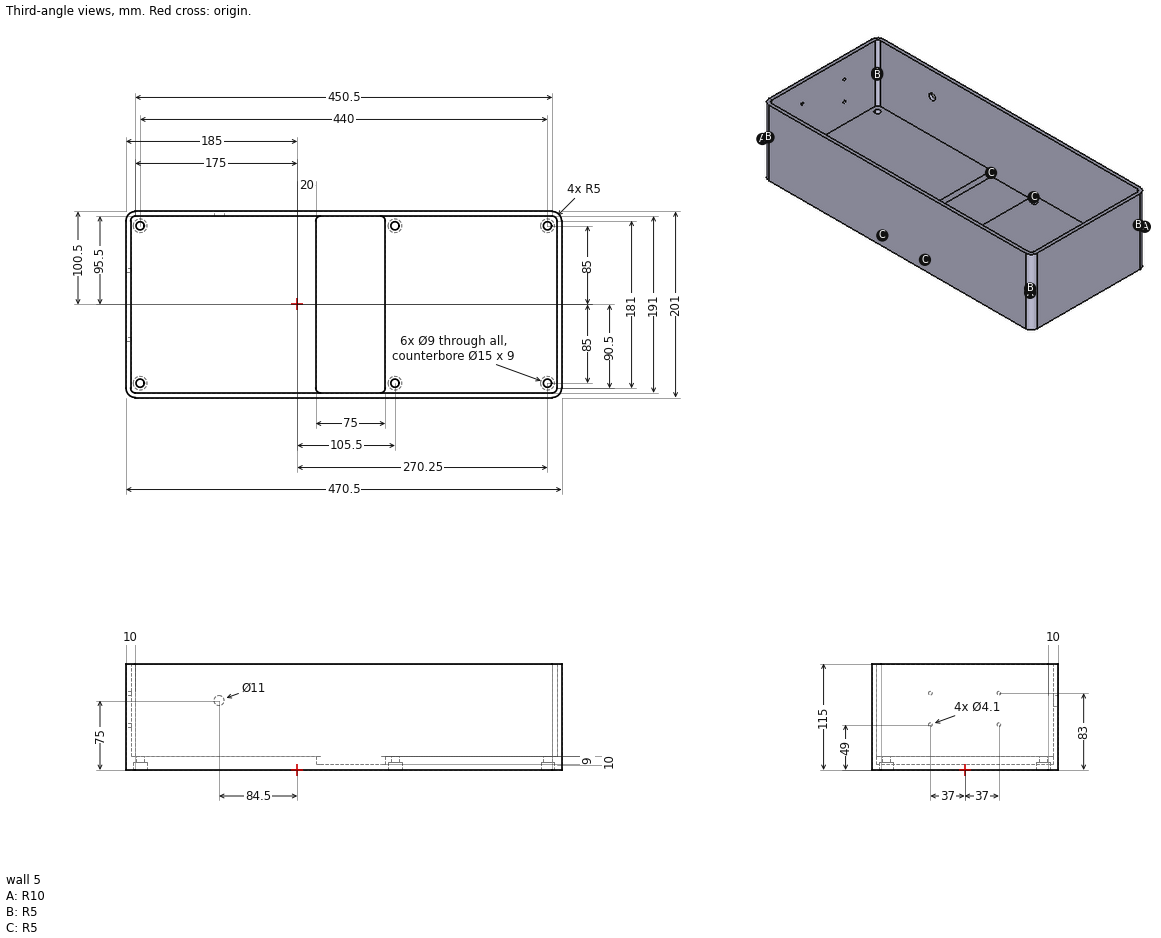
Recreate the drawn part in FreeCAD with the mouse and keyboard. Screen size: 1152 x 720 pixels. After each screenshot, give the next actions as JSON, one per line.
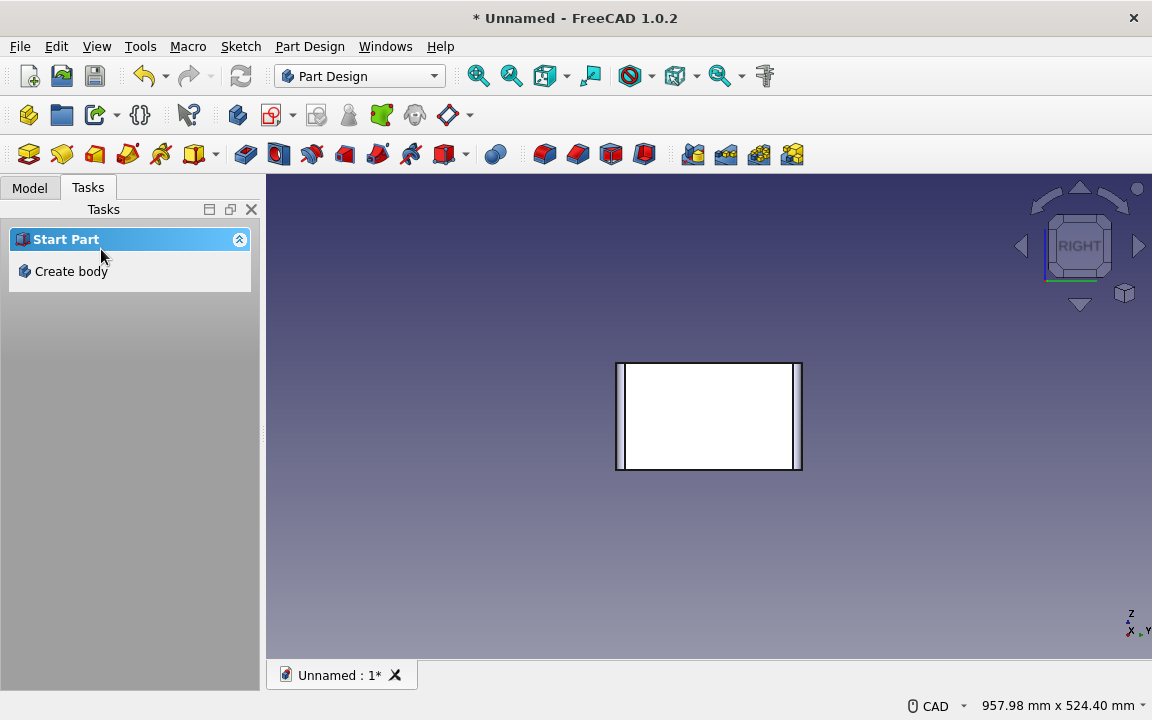
{"action": "key", "text": "5"}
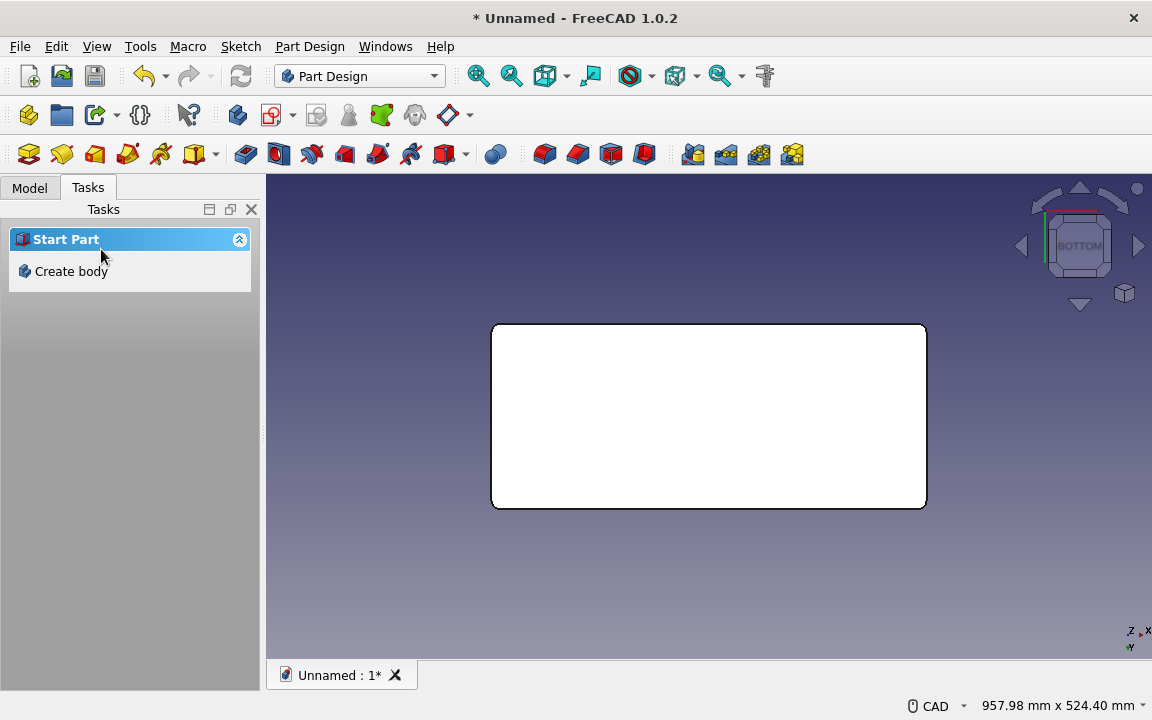
{"action": "key", "text": "4"}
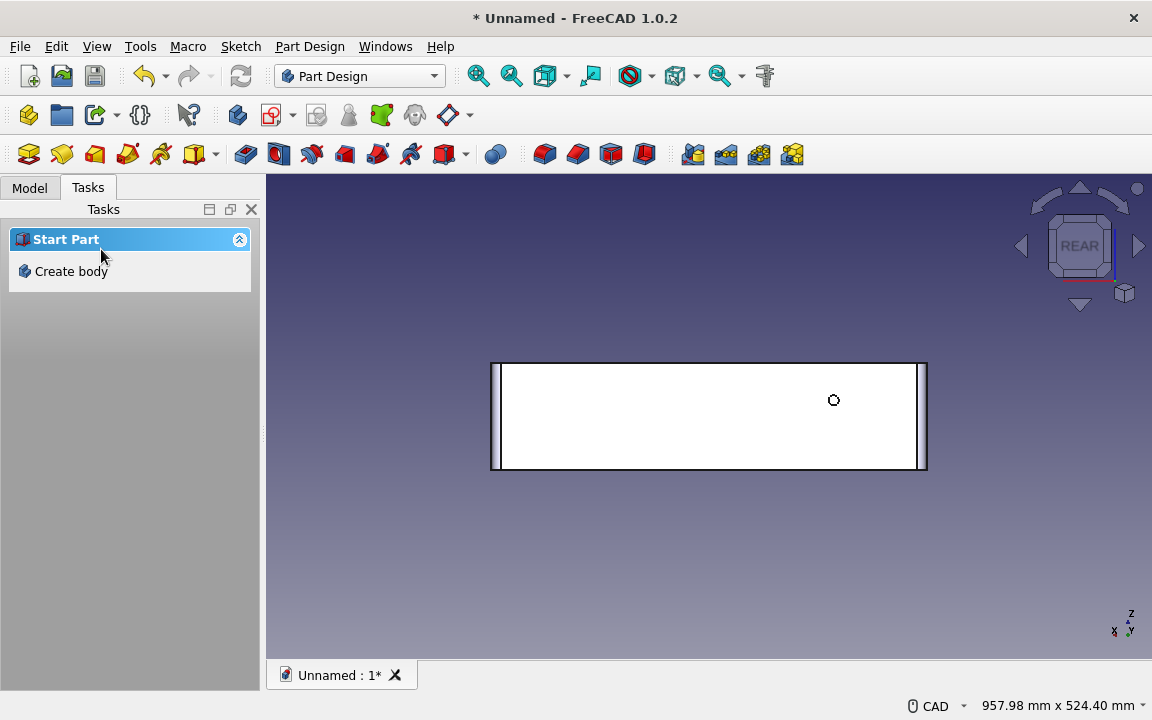
{"action": "key", "text": "6"}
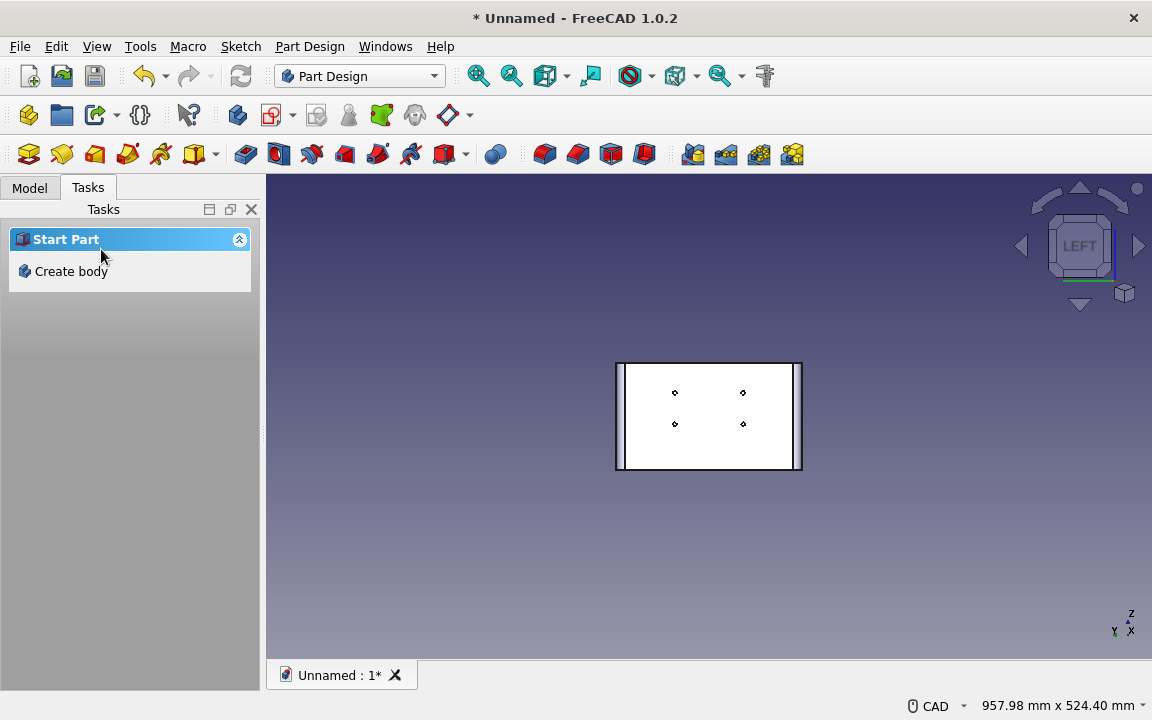
{"action": "key", "text": "v f"}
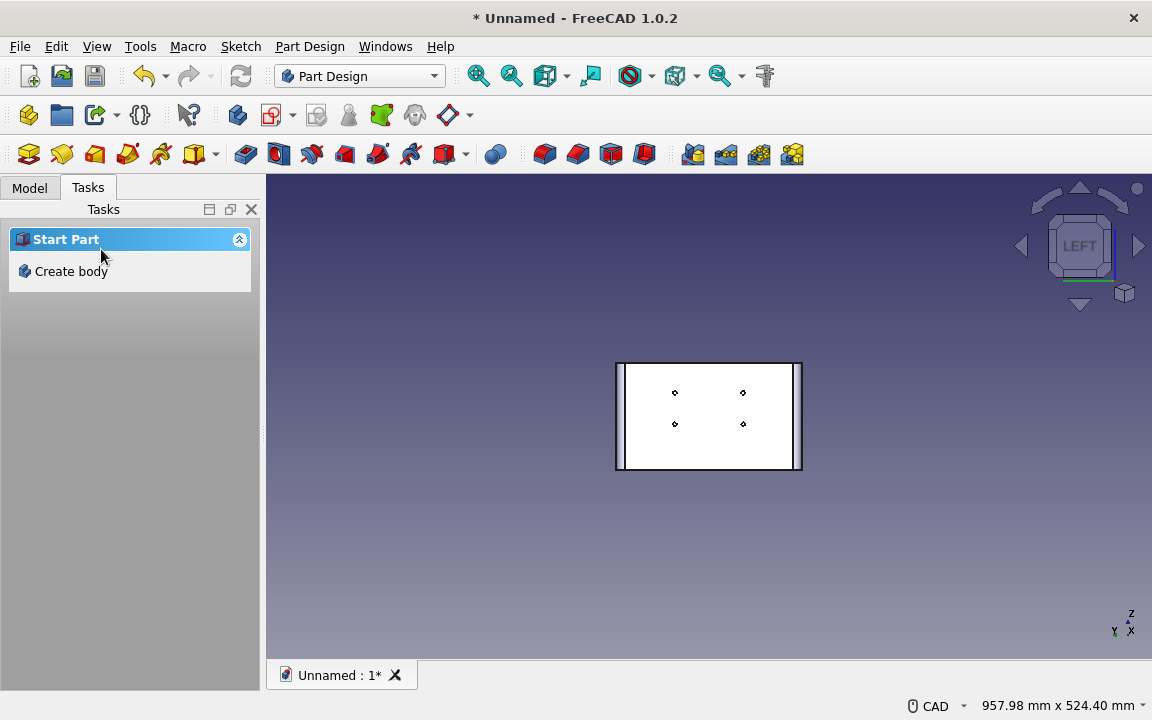
{"action": "key", "text": "v 3"}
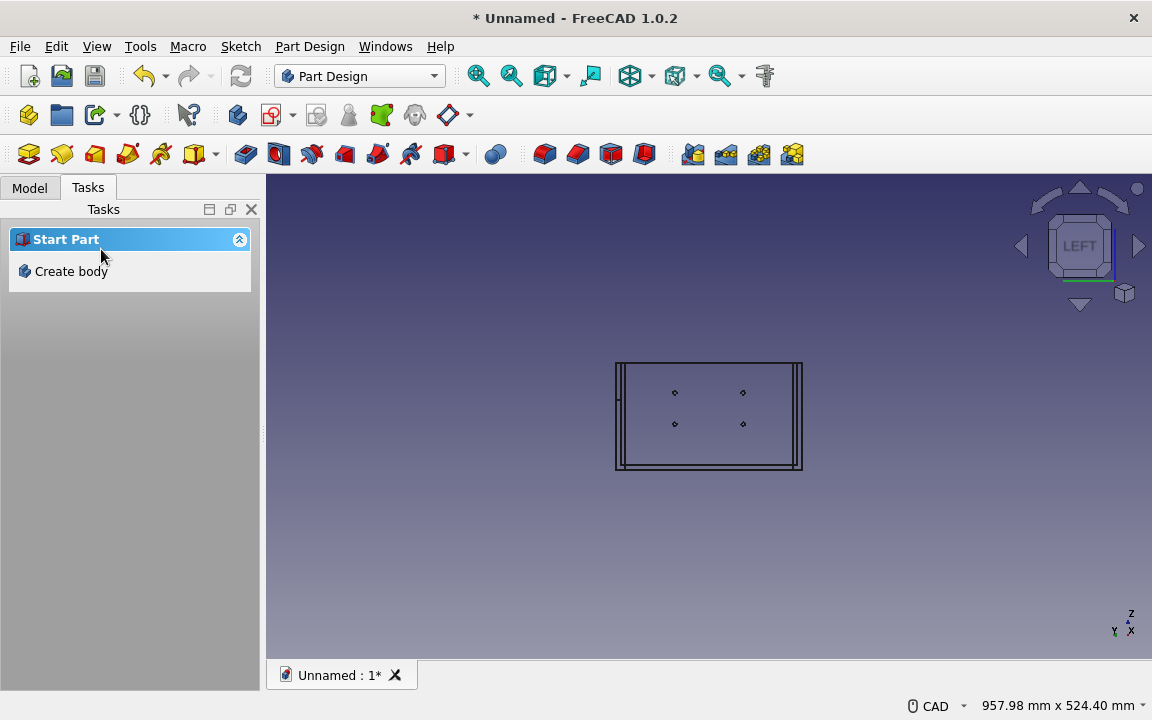
{"action": "key", "text": "0"}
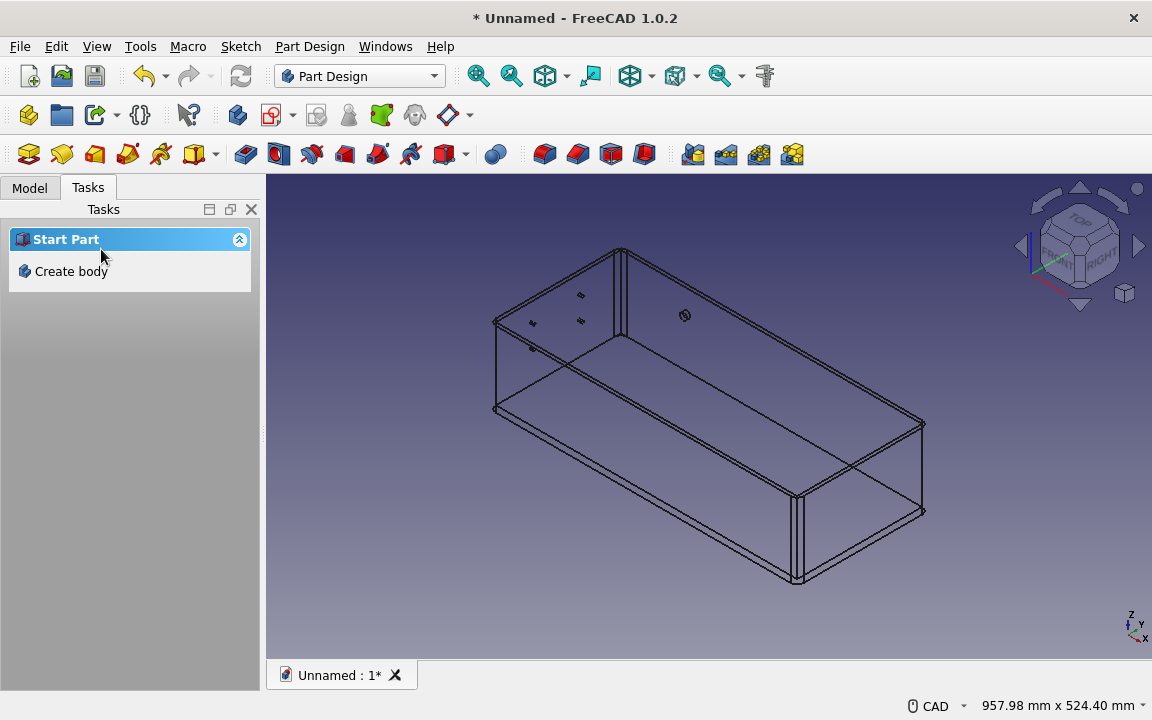
{"action": "left_click", "coordinate": [797, 537]}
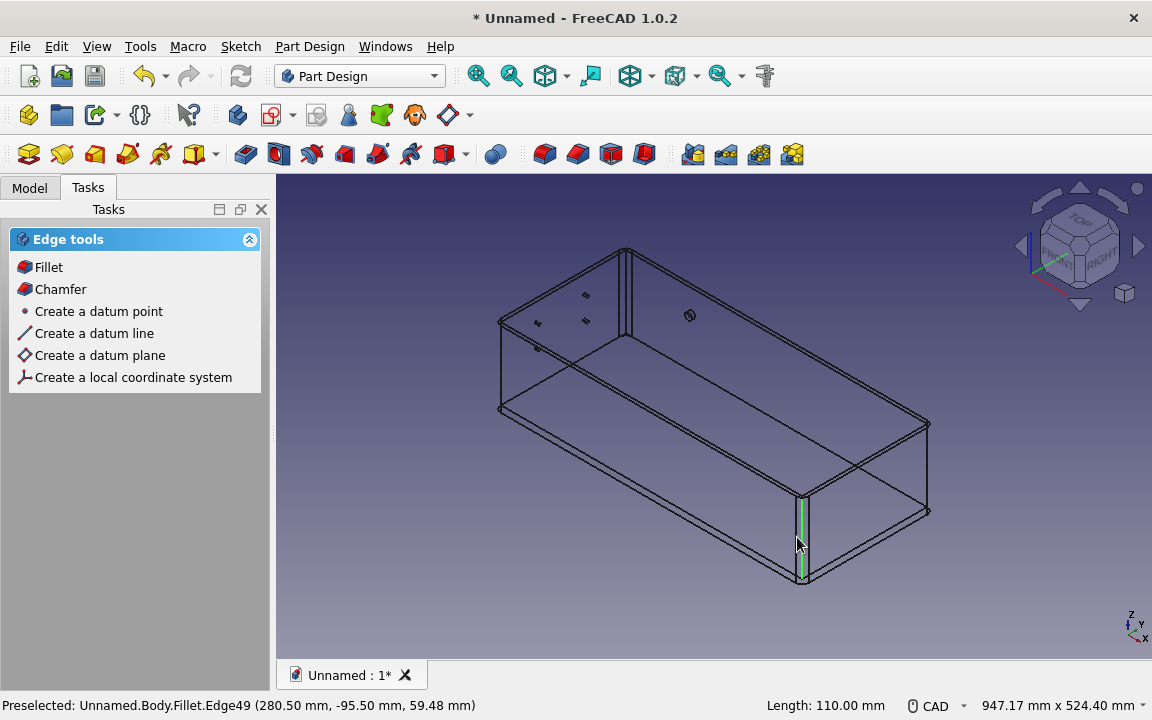
{"action": "left_click", "coordinate": [626, 291], "text": "ctrl"}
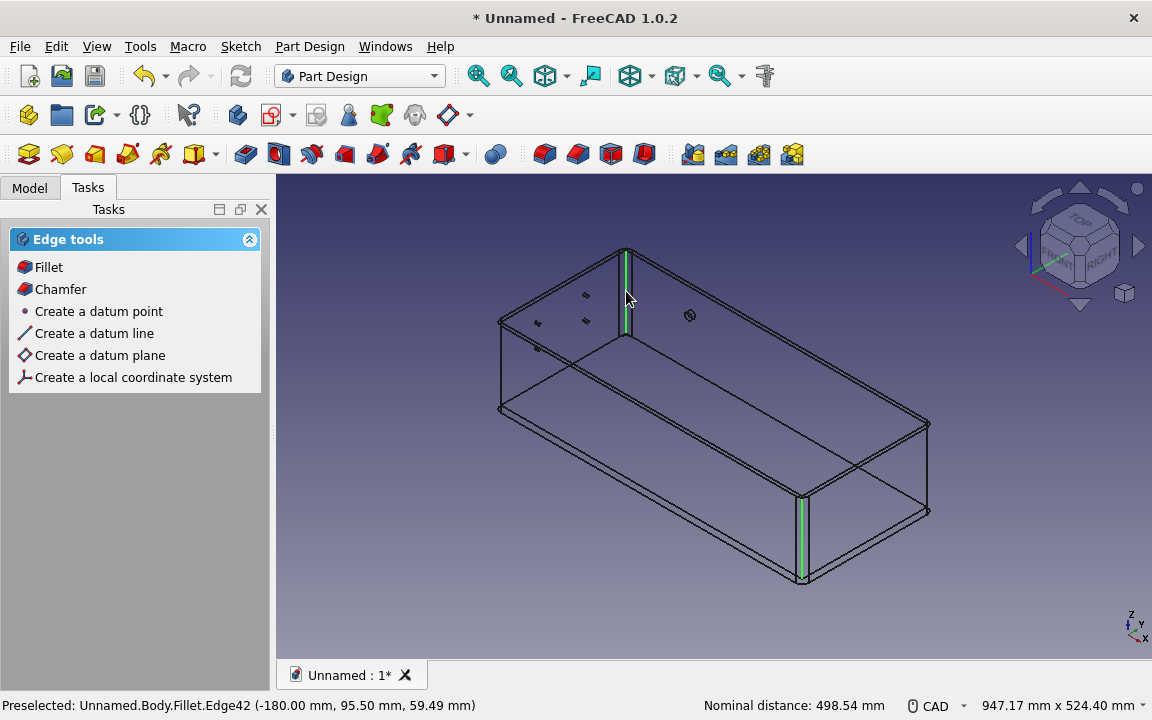
{"action": "scroll", "coordinate": [927, 464], "scroll_direction": "up", "scroll_amount": 6}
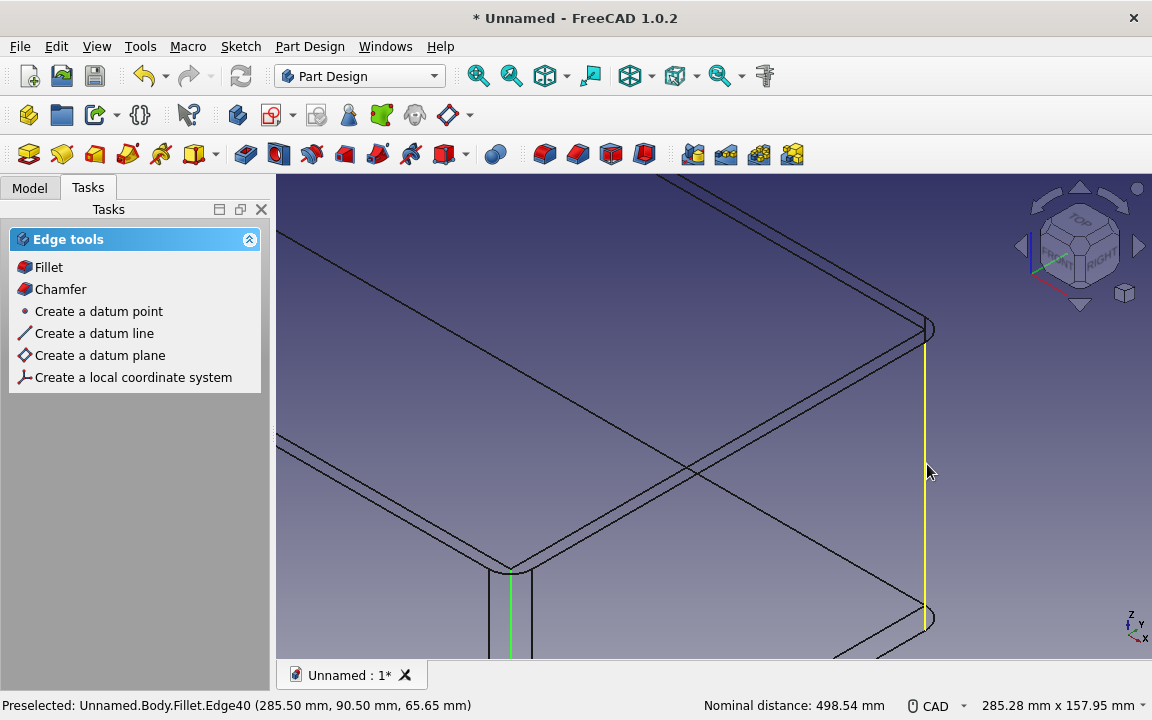
{"action": "left_click", "coordinate": [479, 76]}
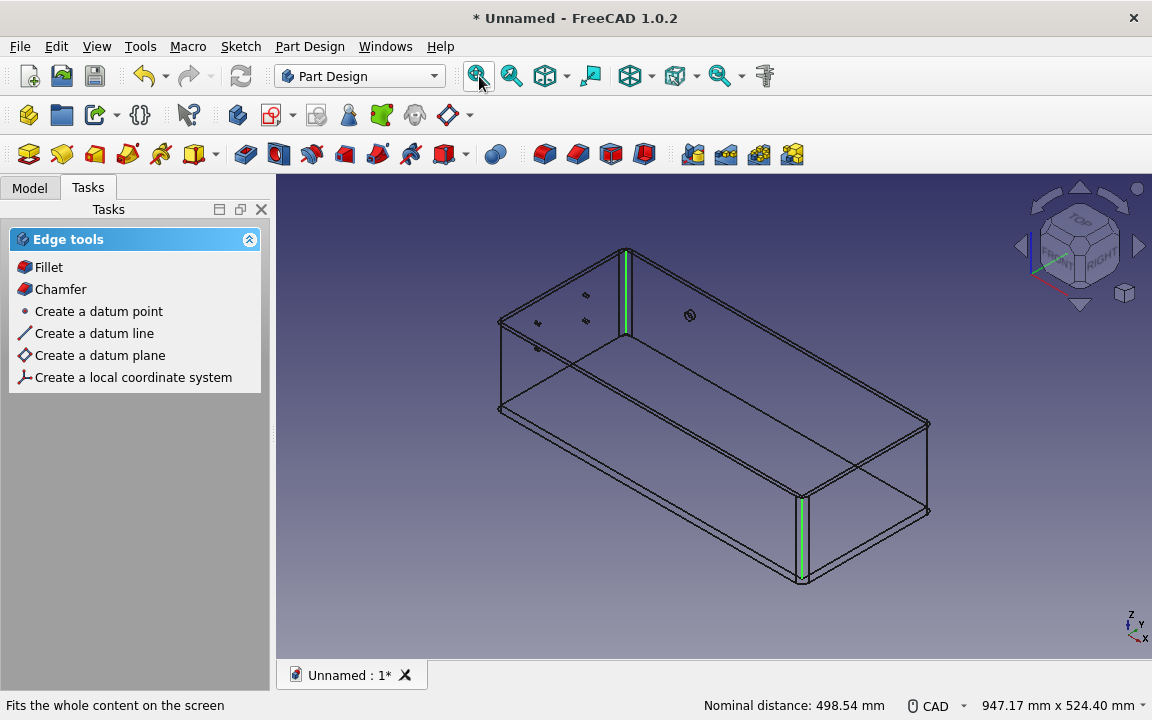
{"action": "key", "text": "2"}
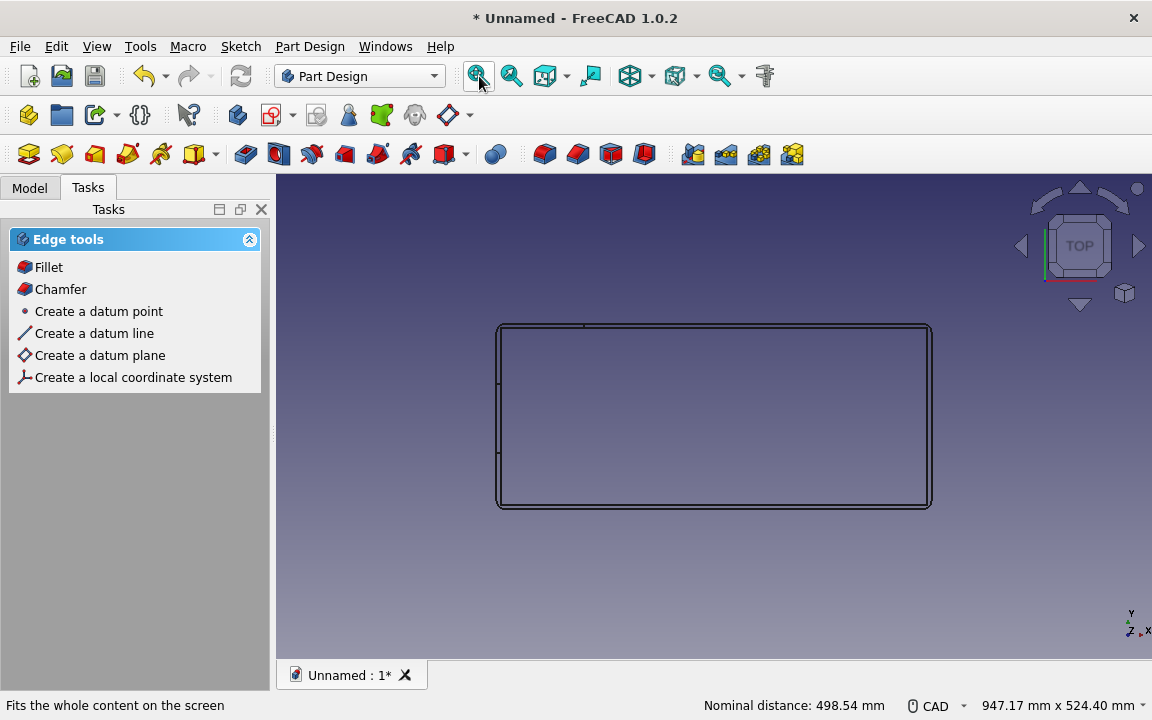
{"action": "scroll", "coordinate": [927, 327], "scroll_direction": "up", "scroll_amount": 6}